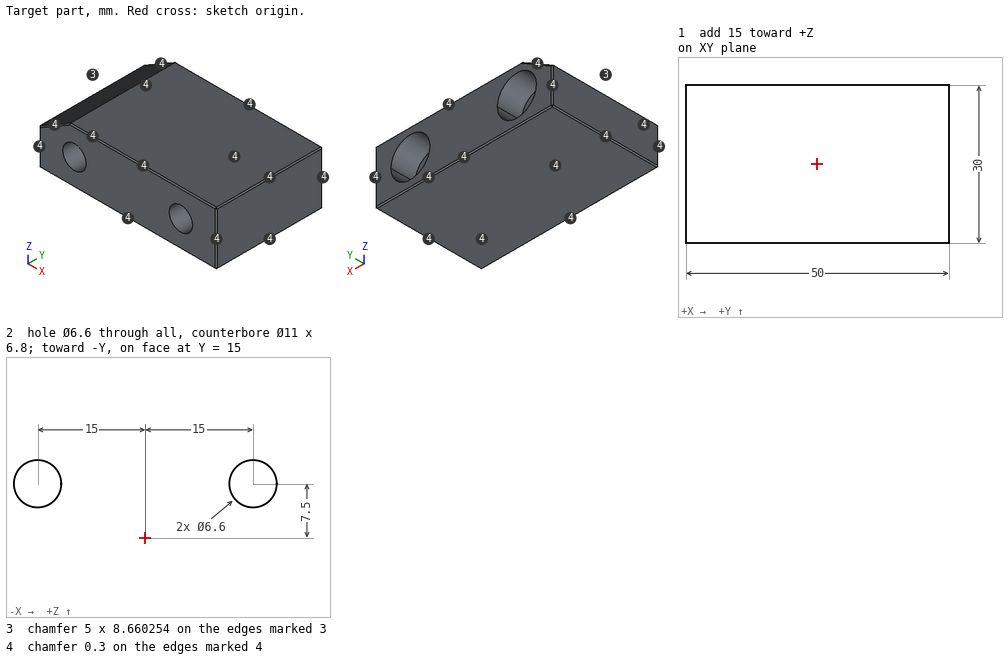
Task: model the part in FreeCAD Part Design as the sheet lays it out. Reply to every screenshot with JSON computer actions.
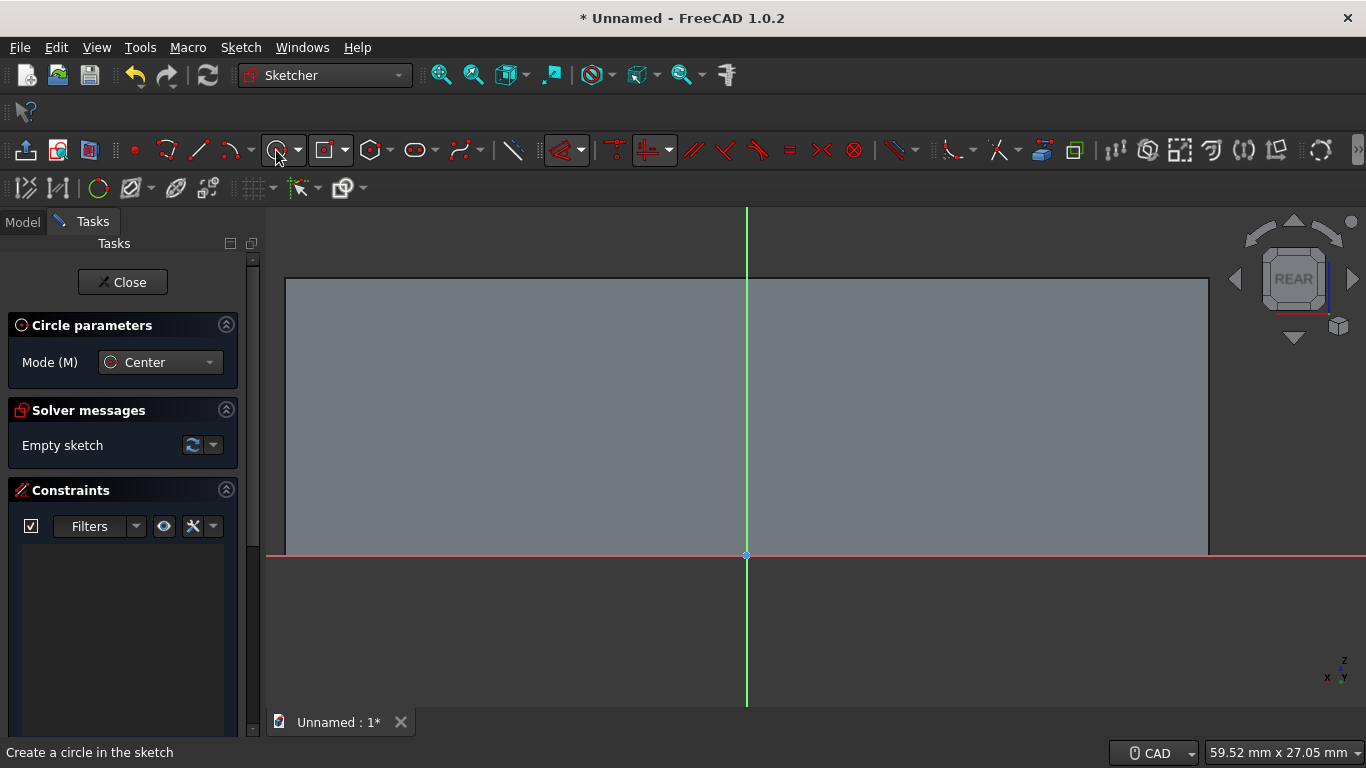
{"action": "left_click", "coordinate": [1024, 417]}
{"action": "mouse_move", "coordinate": [1067, 374]}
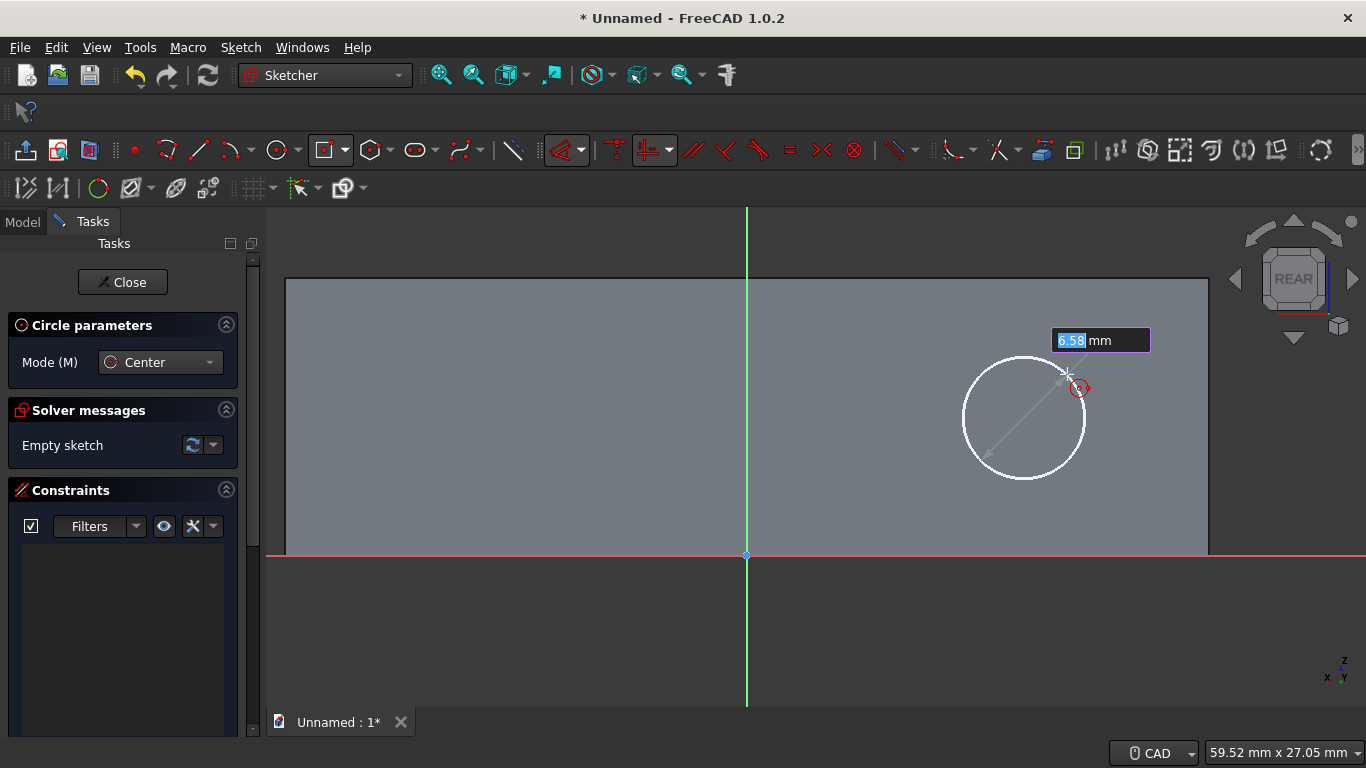
{"action": "type", "text": "6.6"}
{"action": "key", "text": "Return"}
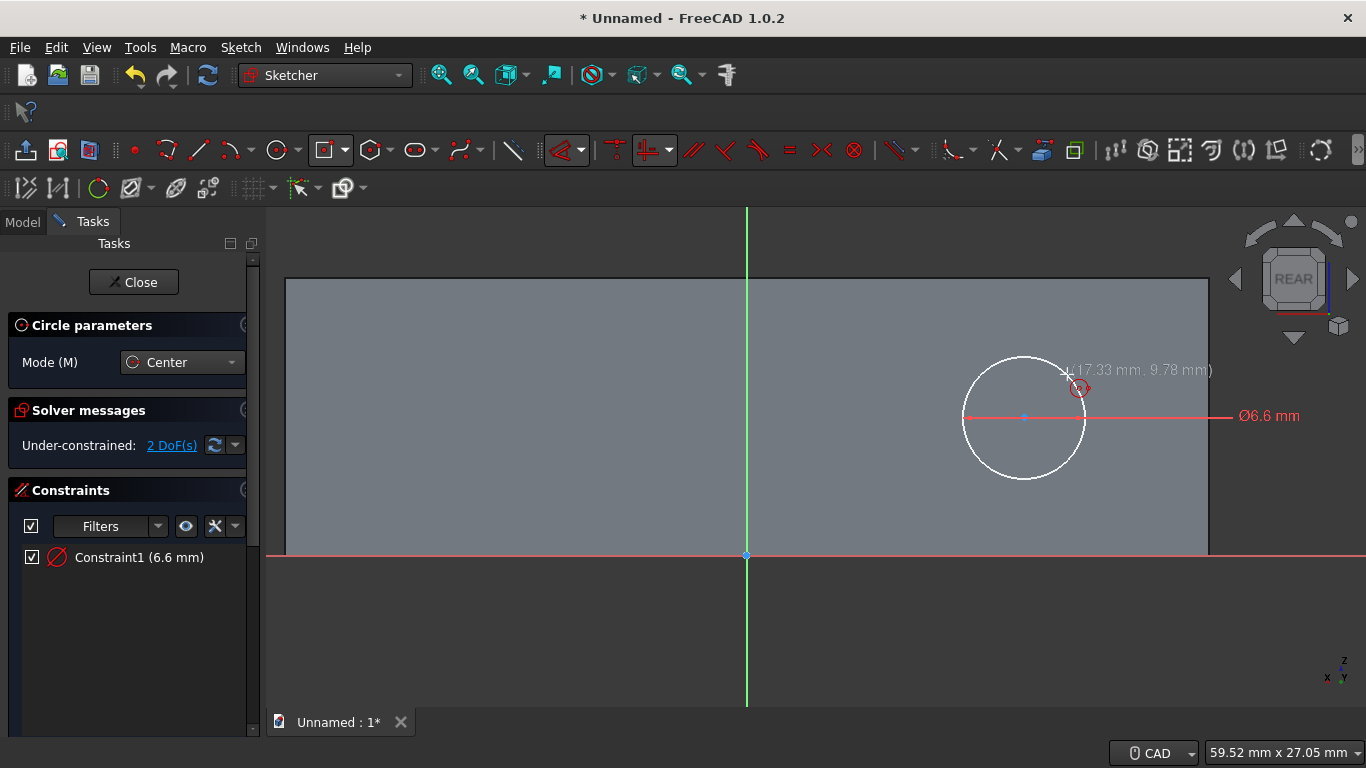
{"action": "left_click", "coordinate": [469, 417]}
{"action": "mouse_move", "coordinate": [513, 374]}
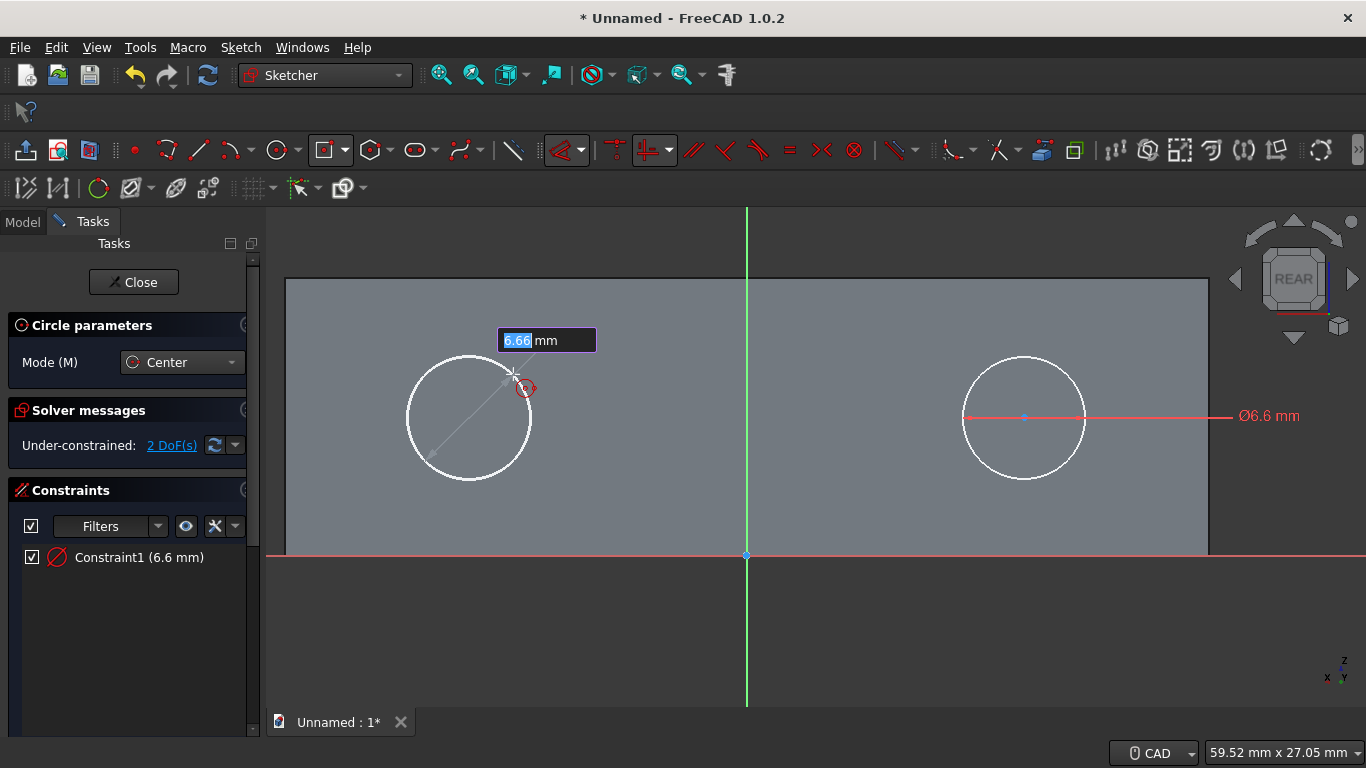
{"action": "type", "text": "6.6"}
{"action": "key", "text": "Return"}
{"action": "key", "text": "Escape"}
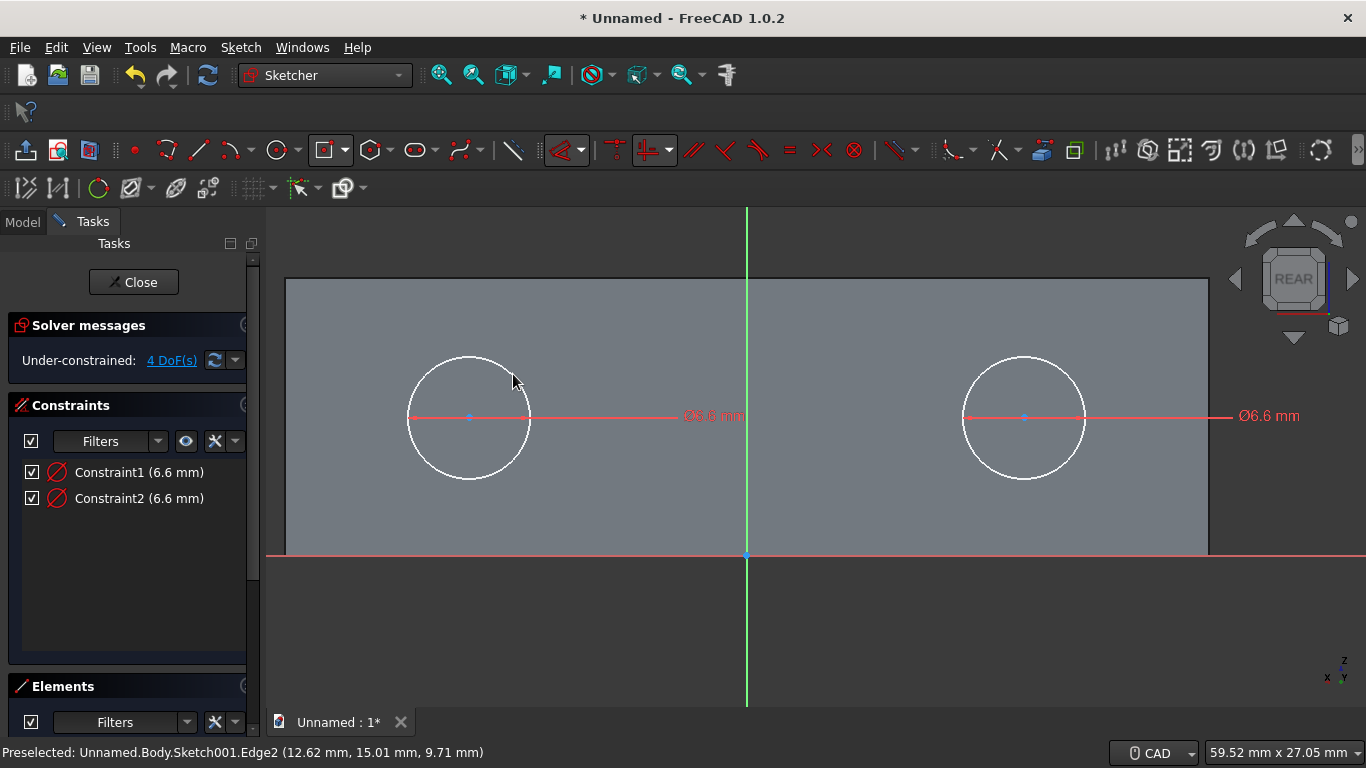
{"action": "left_click", "coordinate": [1024, 418]}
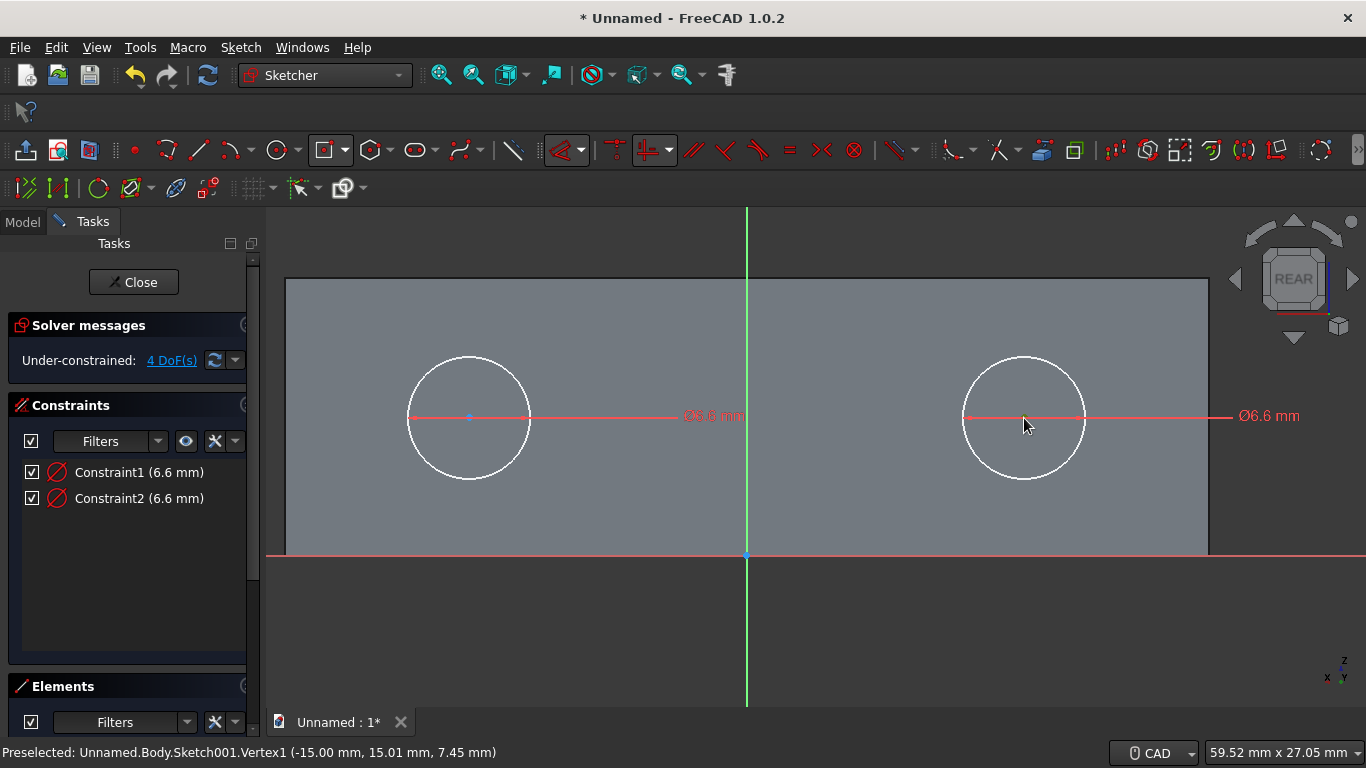
{"action": "left_click", "coordinate": [469, 418]}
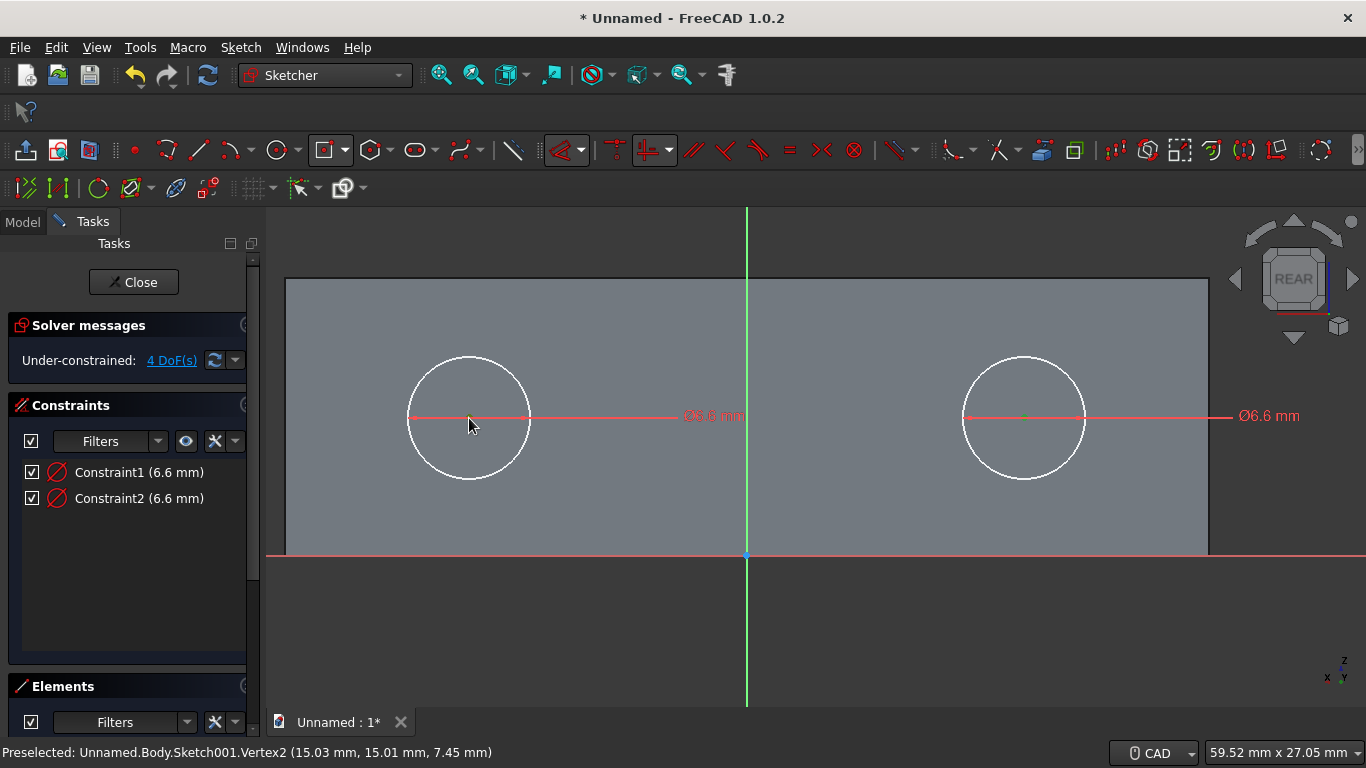
{"action": "key", "text": "h"}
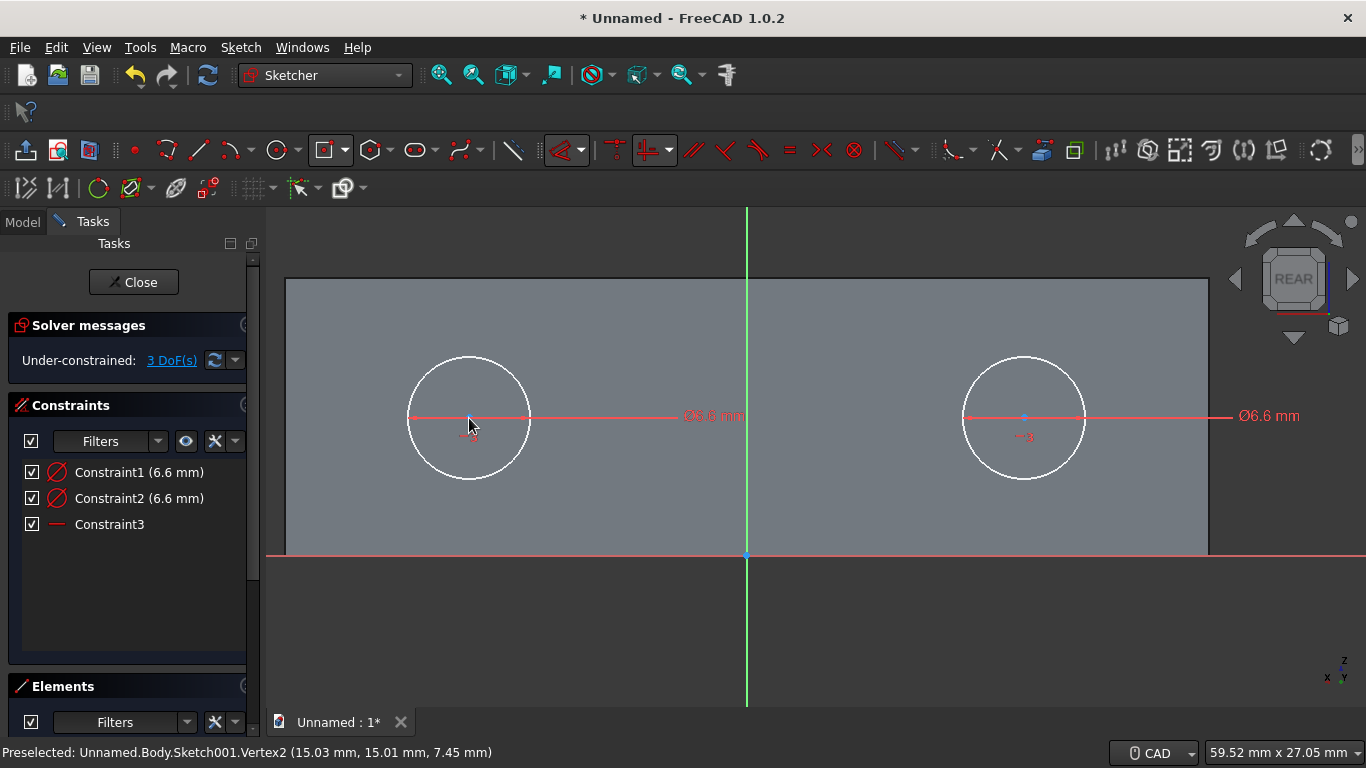
{"action": "left_click", "coordinate": [560, 150]}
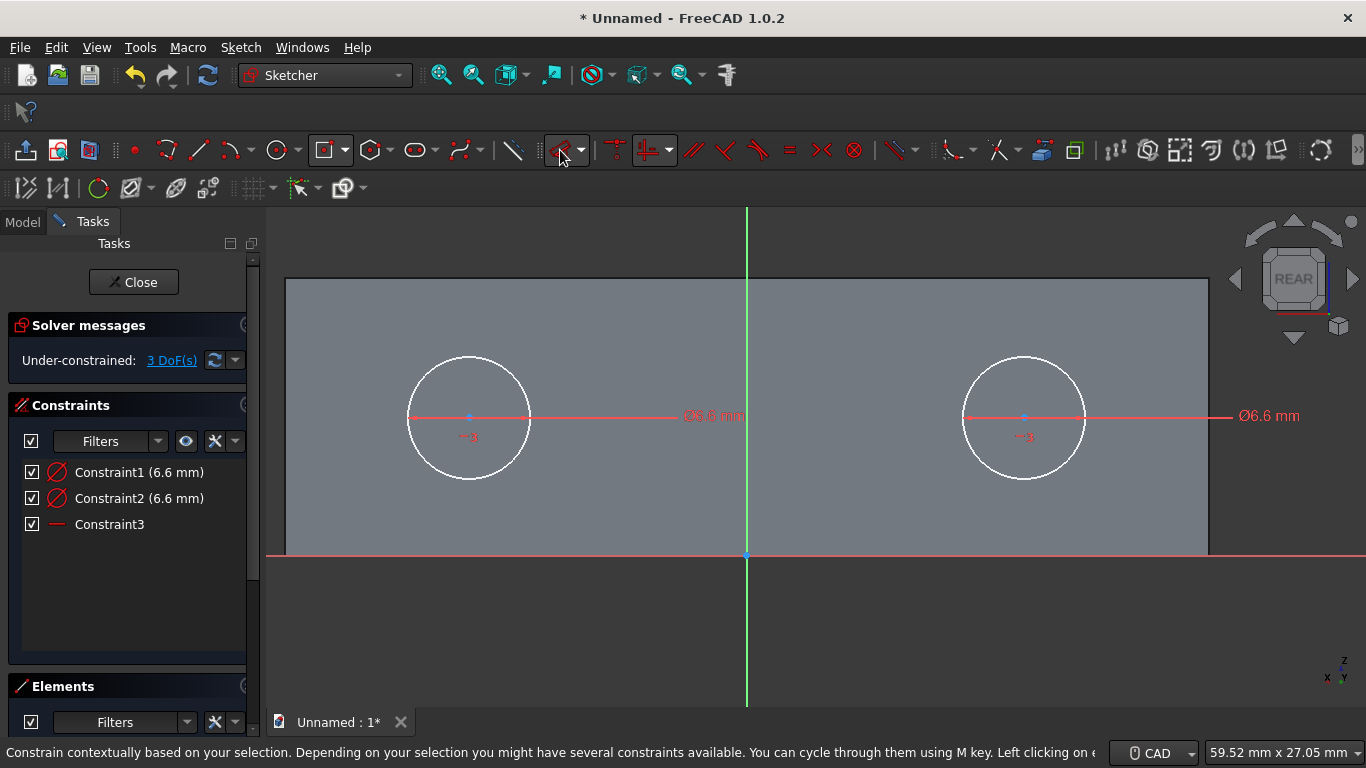
{"action": "left_click", "coordinate": [1024, 418]}
{"action": "left_click", "coordinate": [885, 590]}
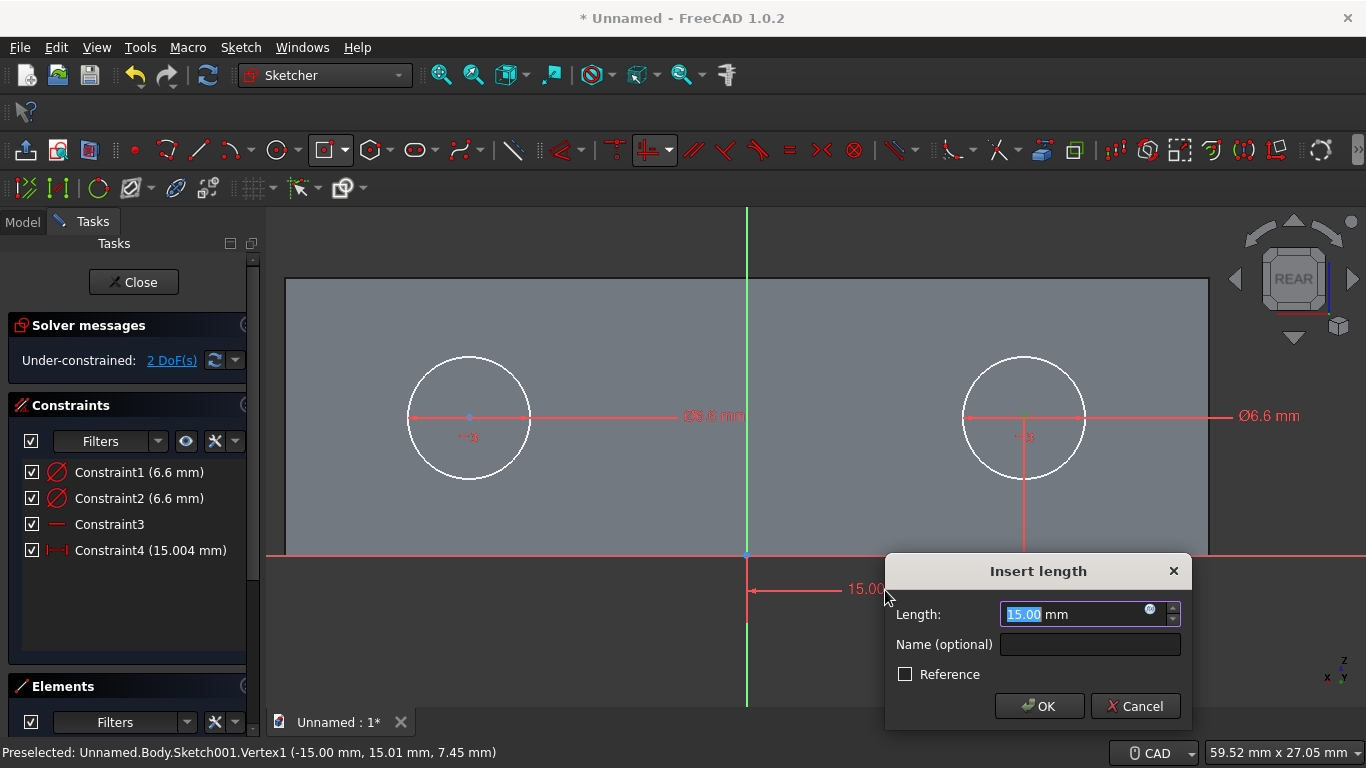
{"action": "type", "text": "15"}
{"action": "key", "text": "Return"}